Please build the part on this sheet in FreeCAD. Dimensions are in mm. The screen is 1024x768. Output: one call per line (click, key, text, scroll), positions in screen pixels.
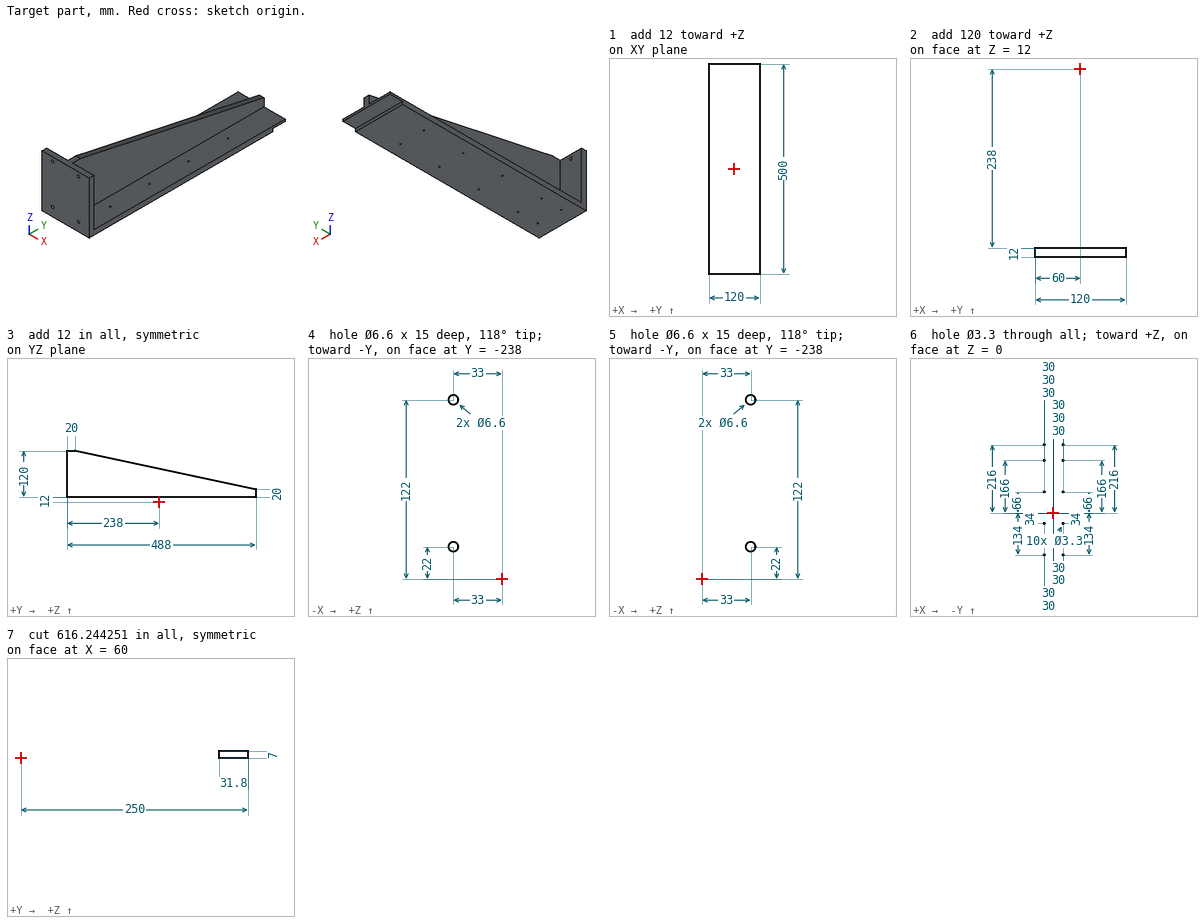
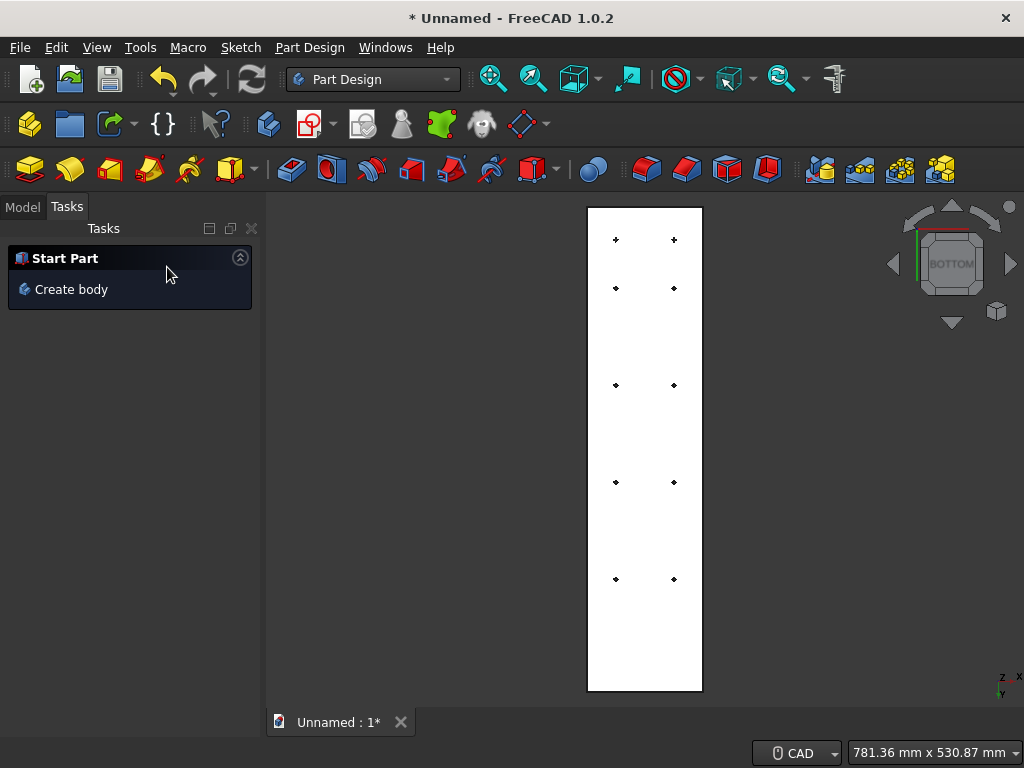
key(0)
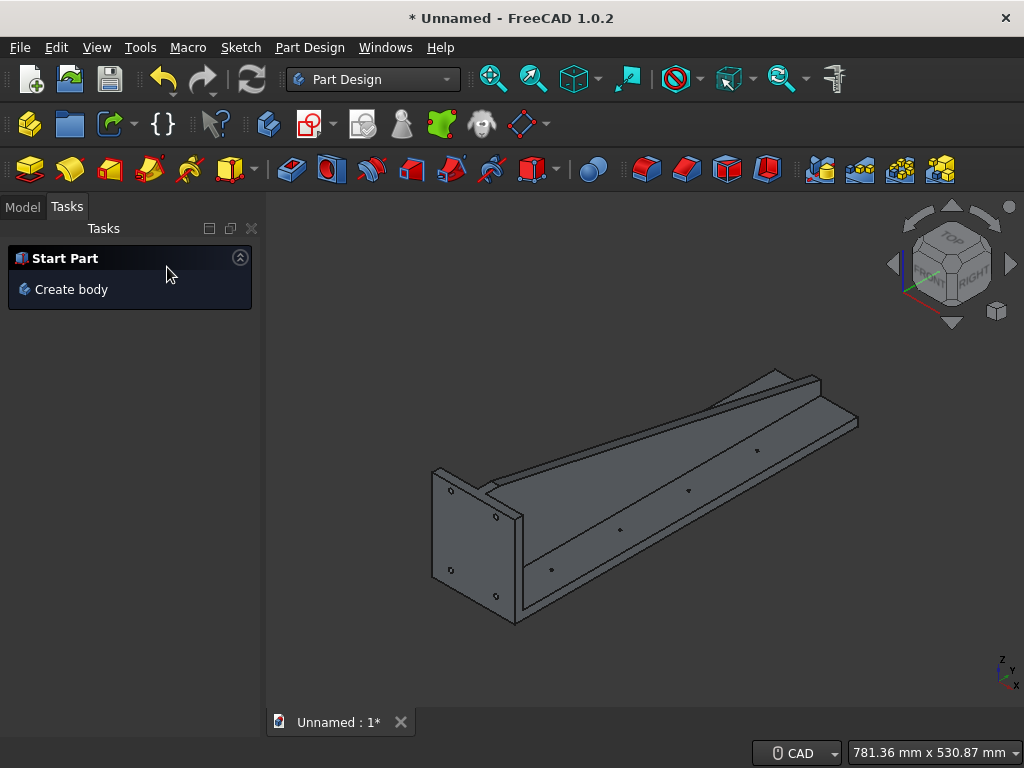
scroll(833, 432, up, 8)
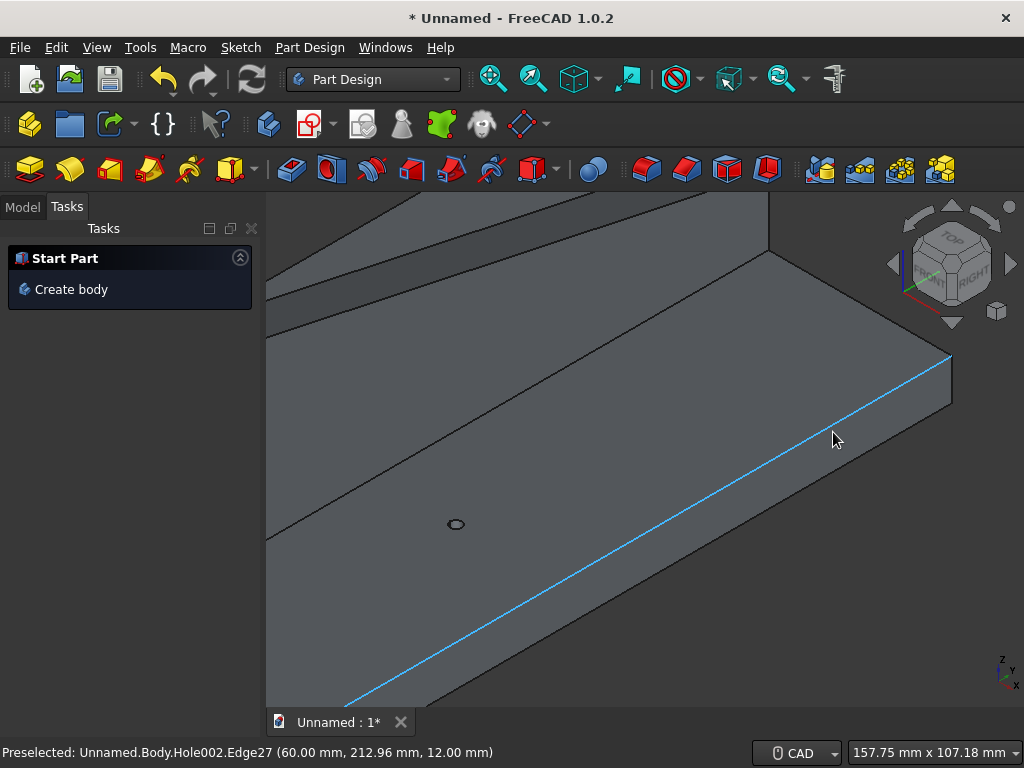
click(494, 80)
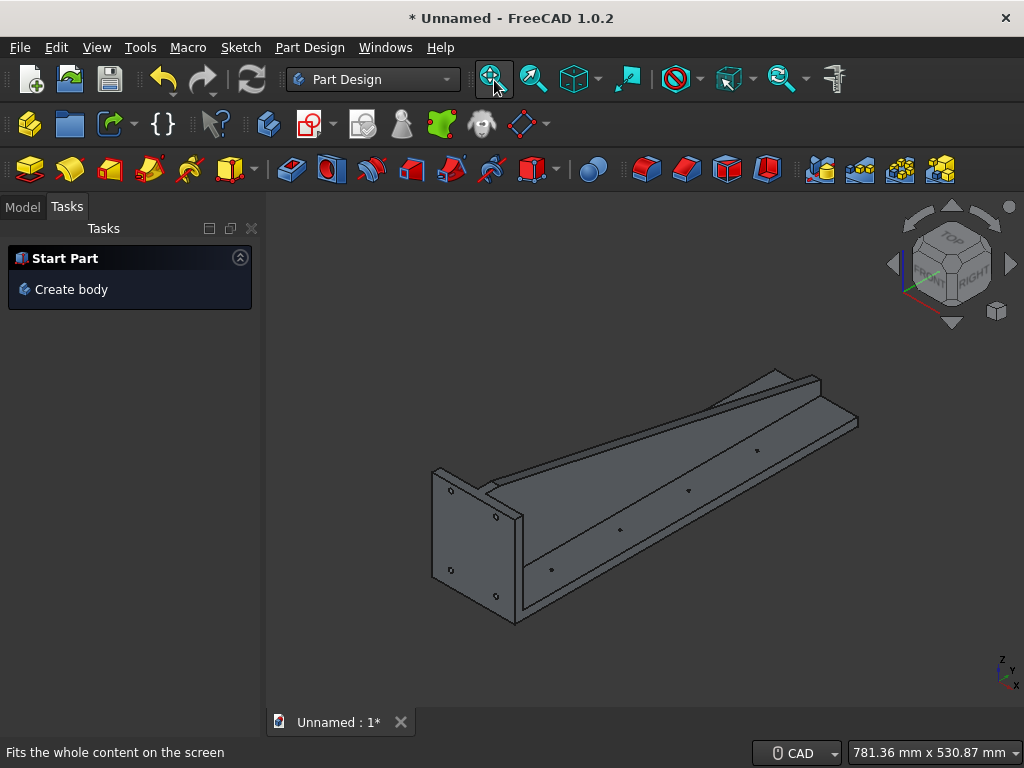
key(3)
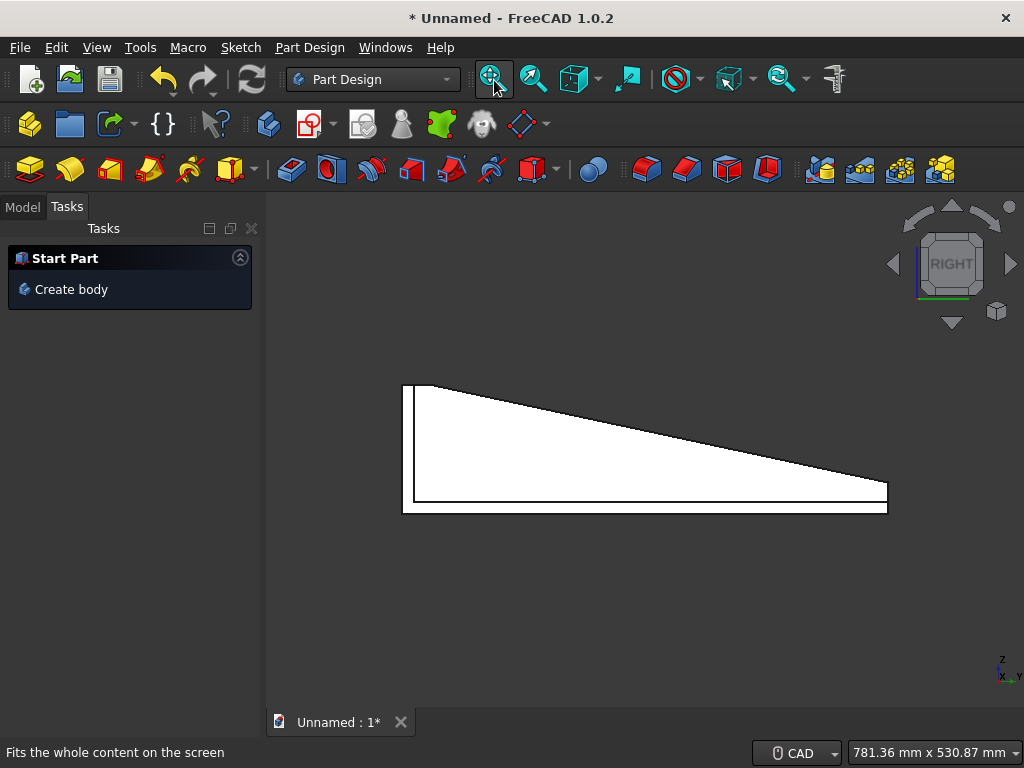
scroll(853, 503, up, 8)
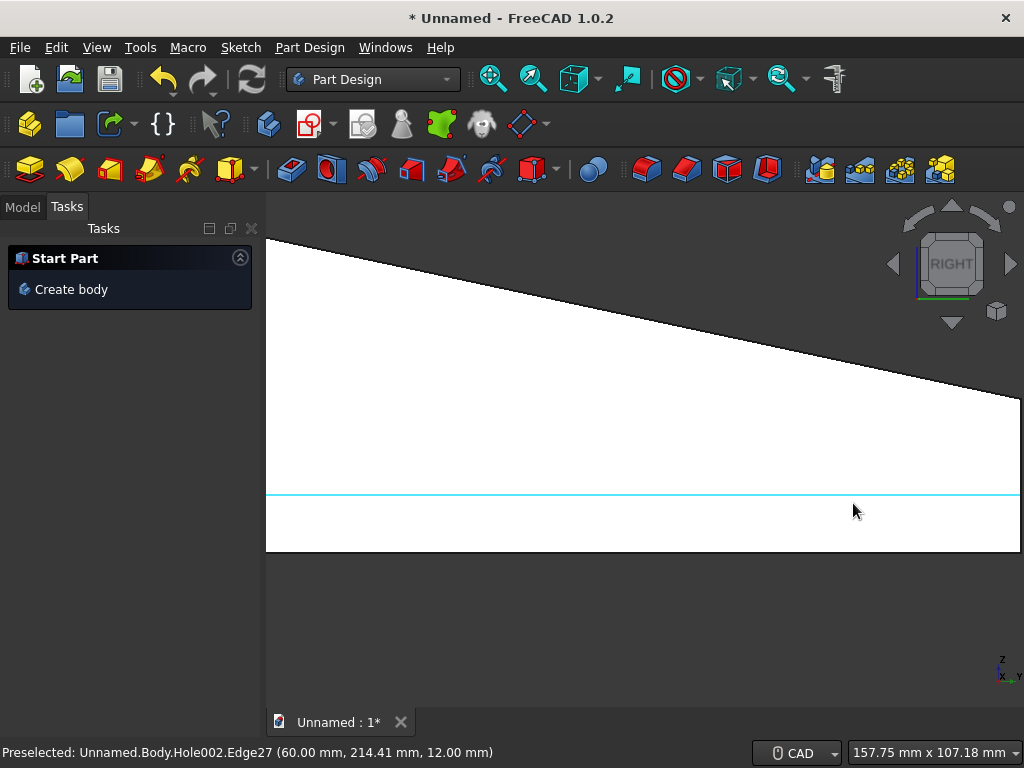
click(849, 506)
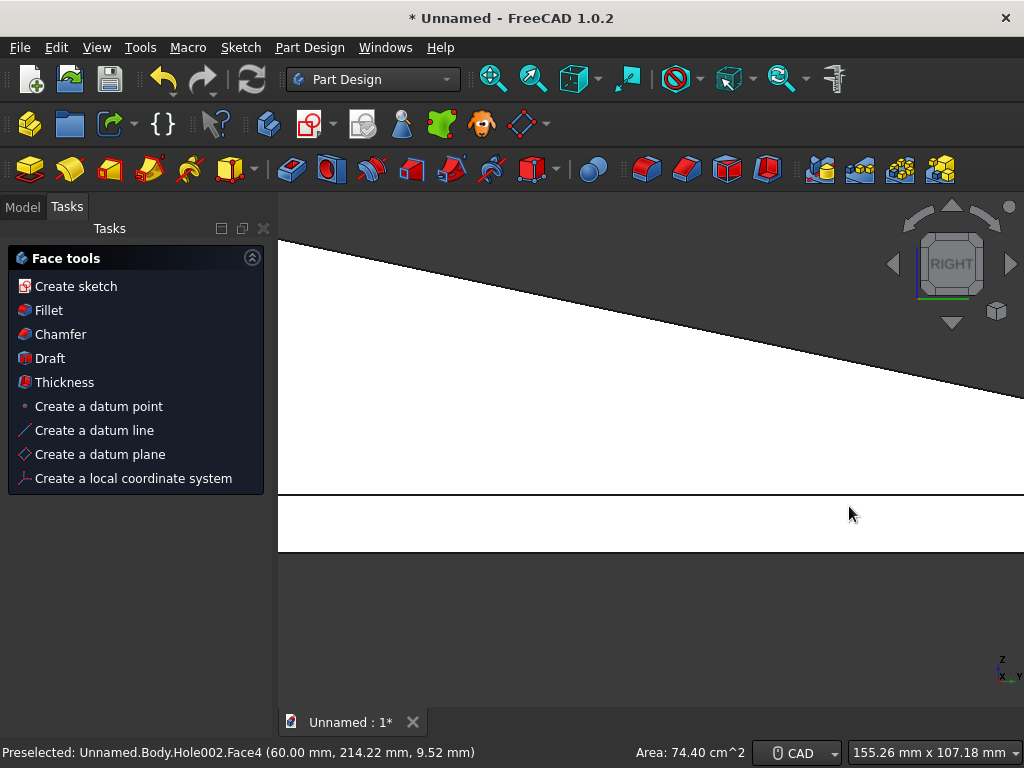
click(310, 124)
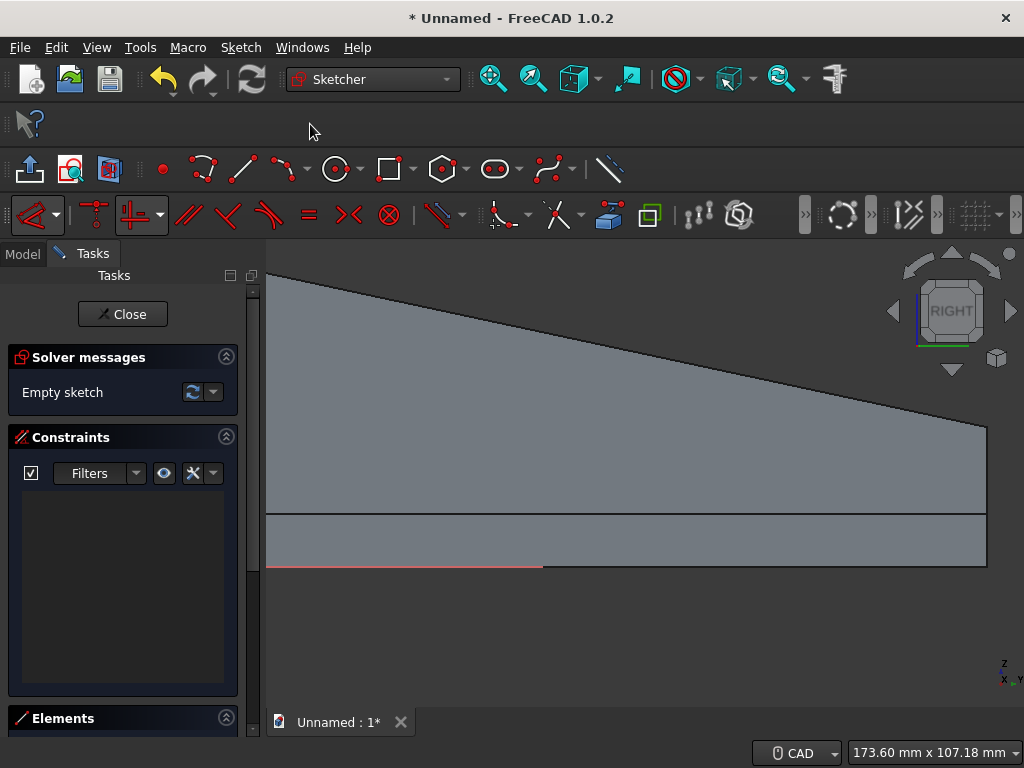
scroll(576, 473, down, 5)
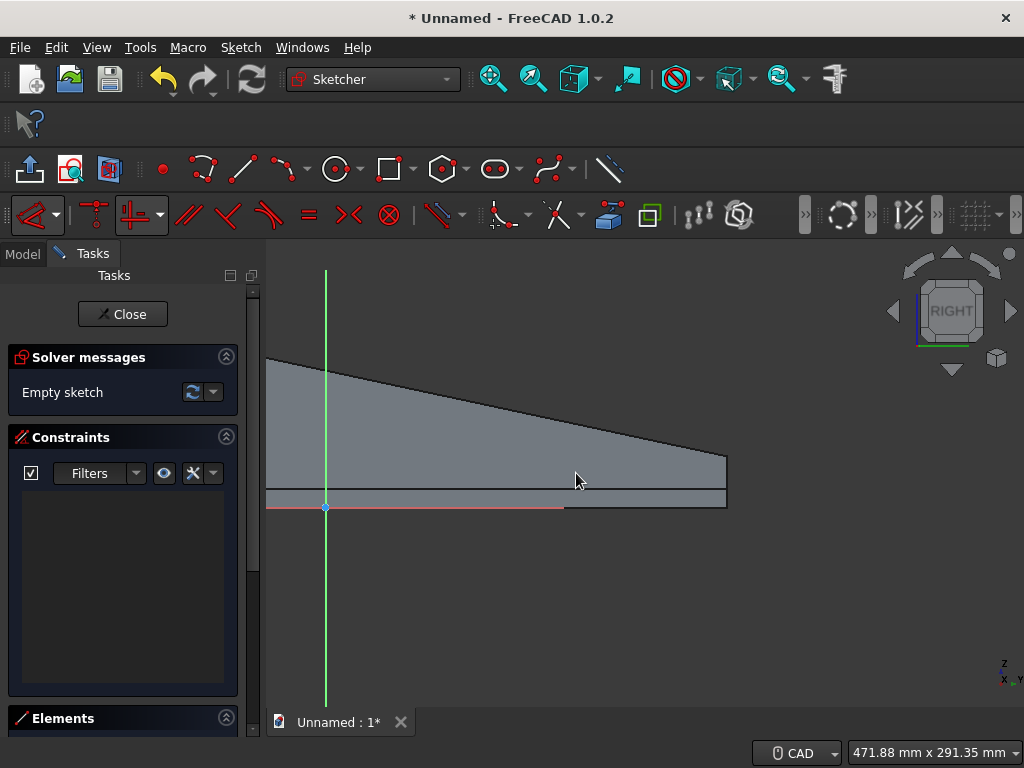
scroll(721, 507, up, 10)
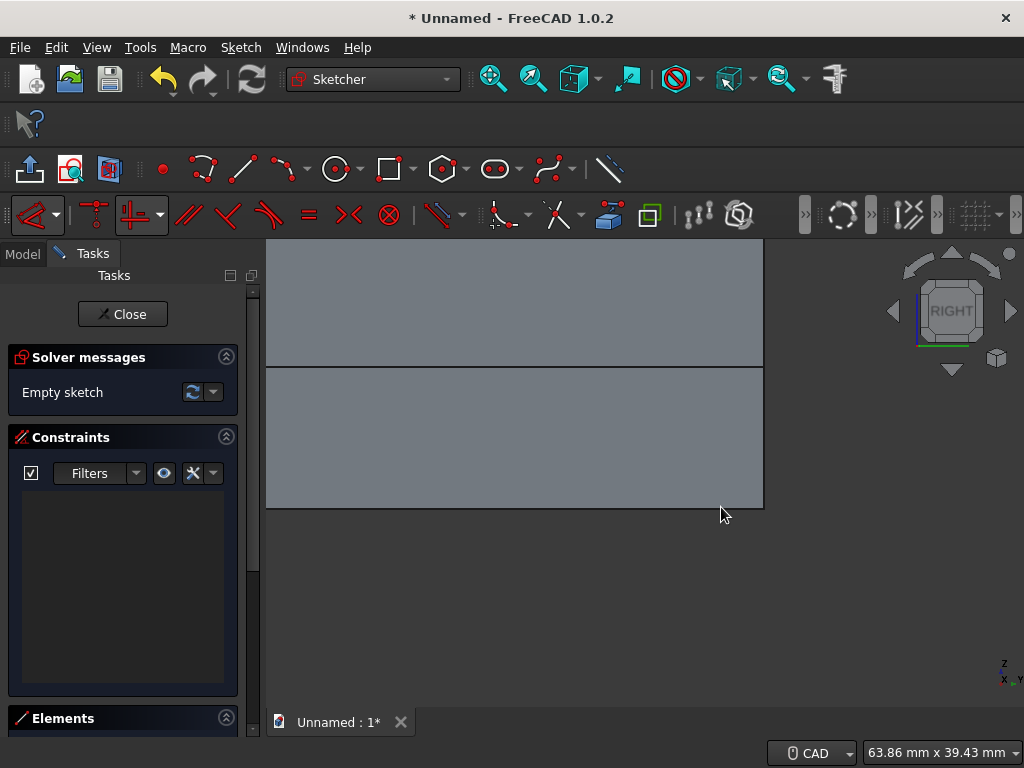
click(390, 170)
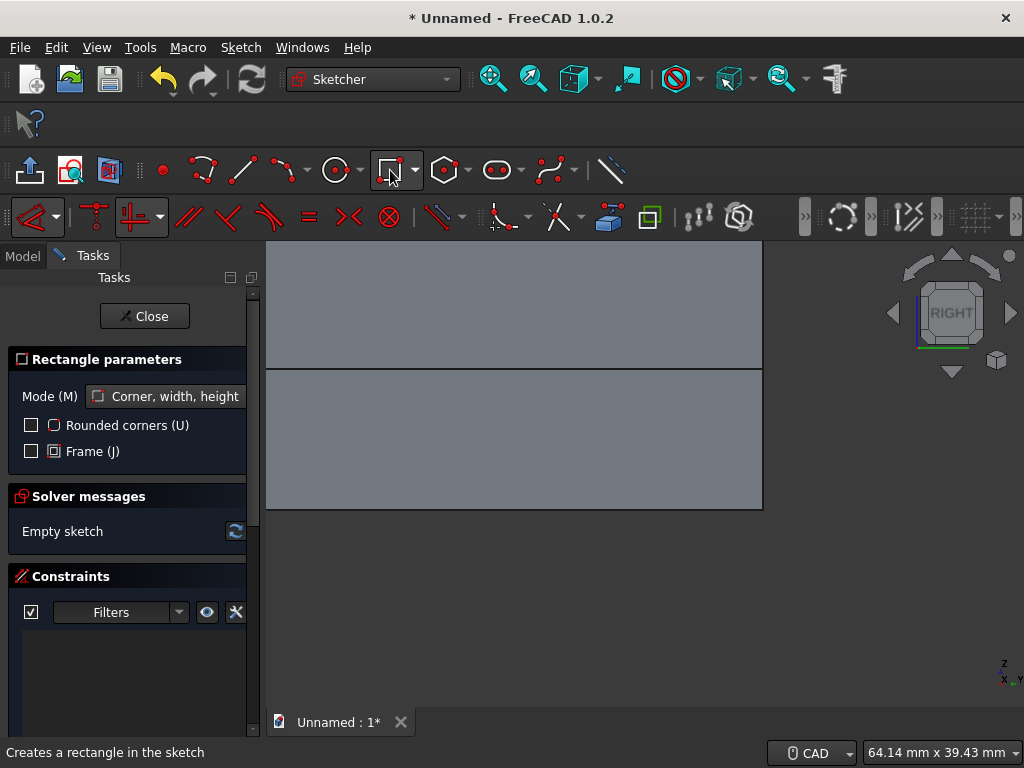
click(388, 428)
click(763, 510)
key(Escape)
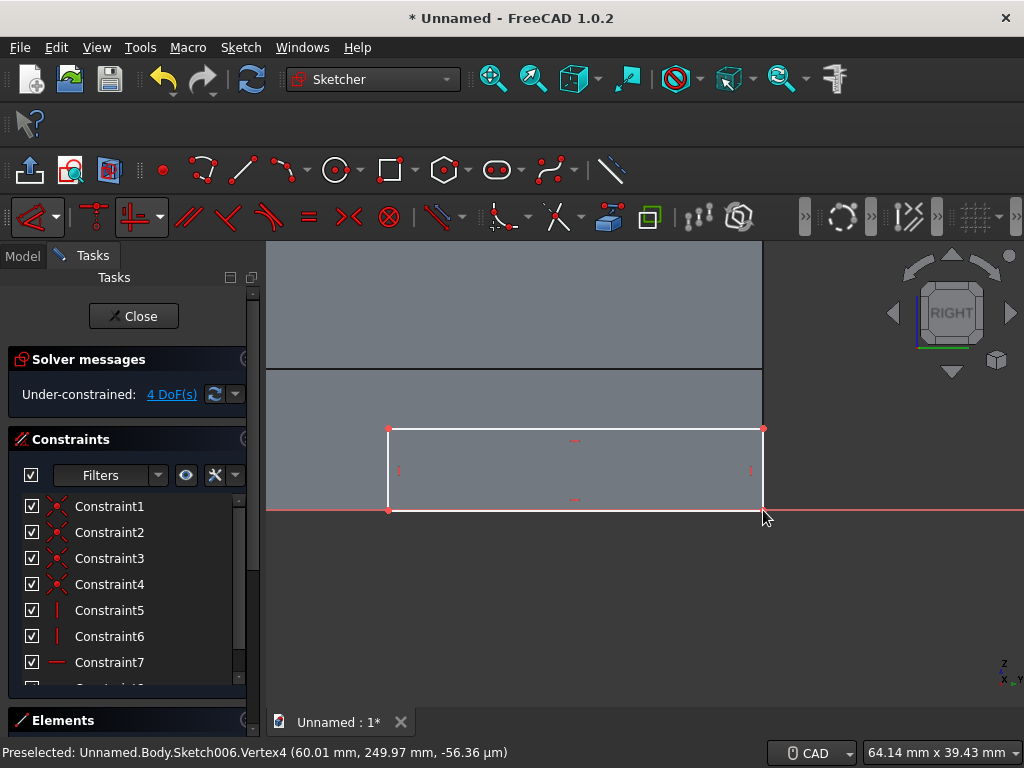
click(388, 511)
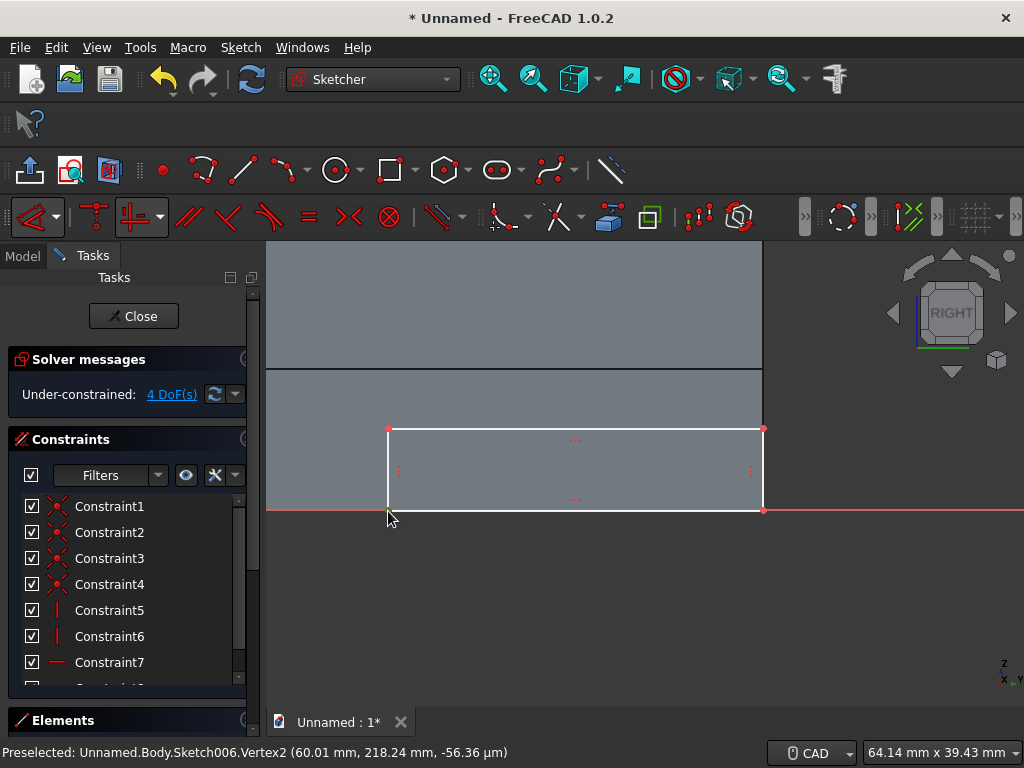
click(334, 510)